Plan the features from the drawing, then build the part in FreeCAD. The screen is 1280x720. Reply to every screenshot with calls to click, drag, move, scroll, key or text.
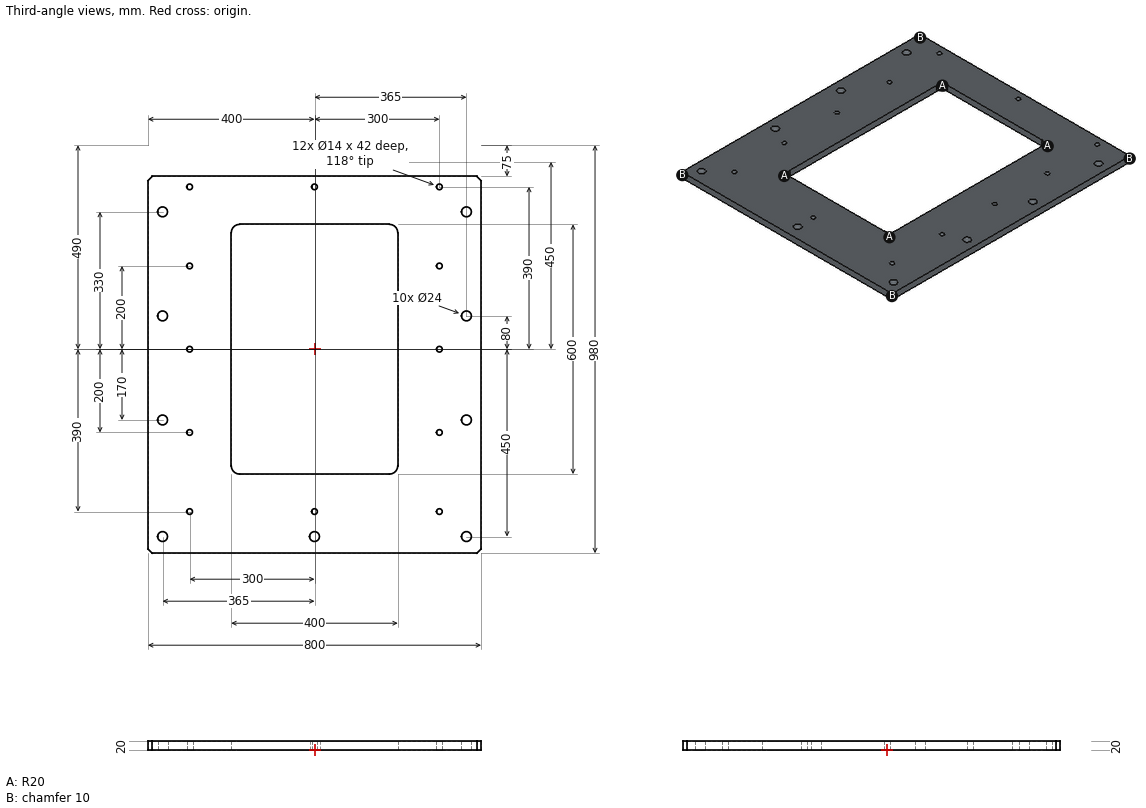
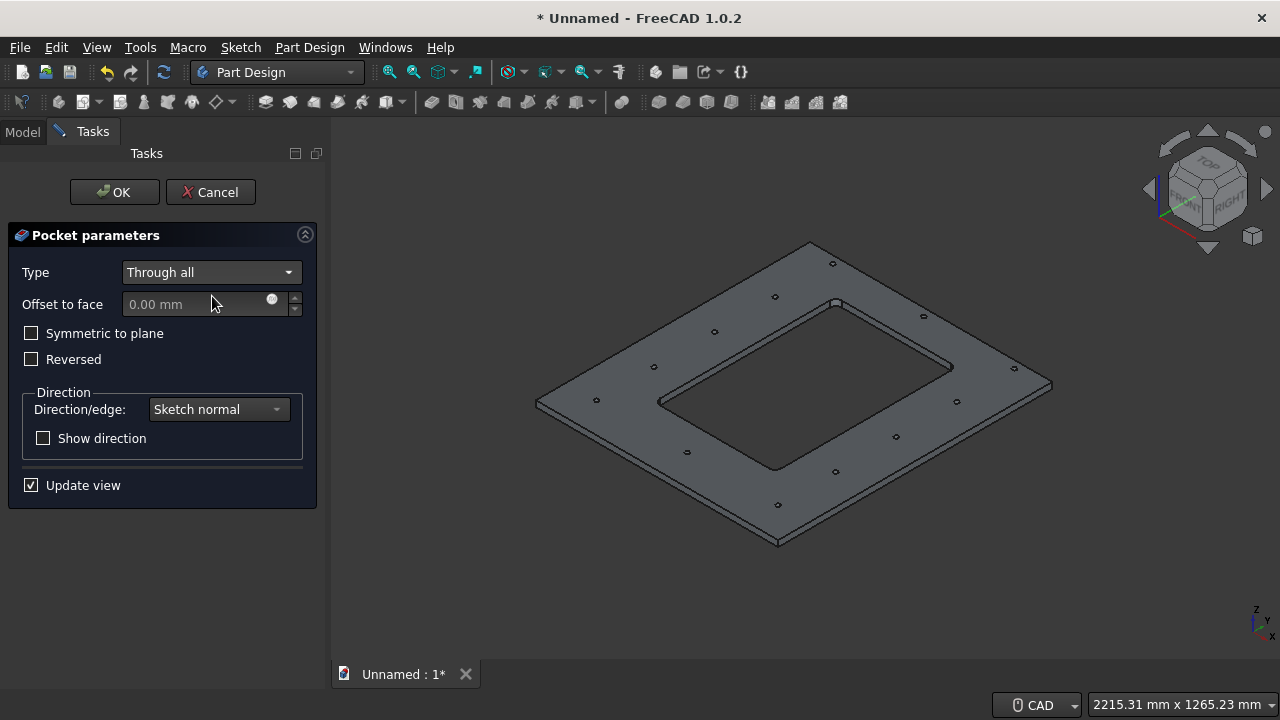
click(115, 192)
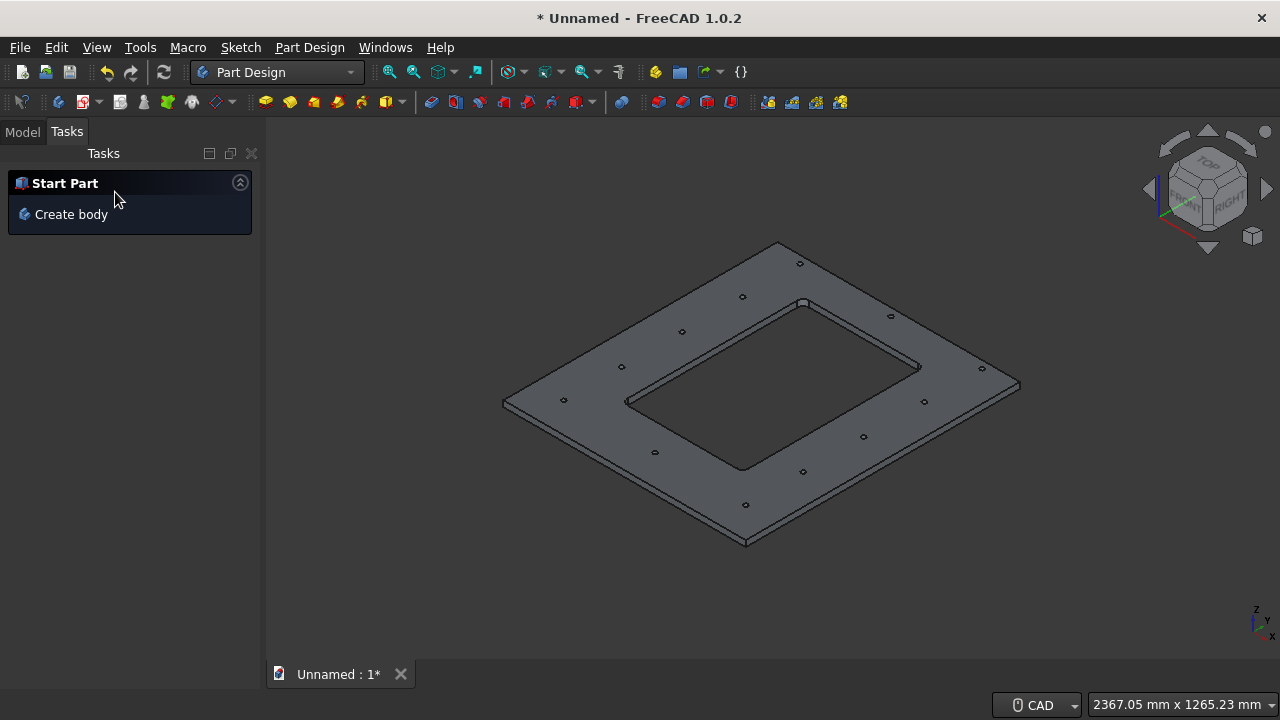
click(948, 362)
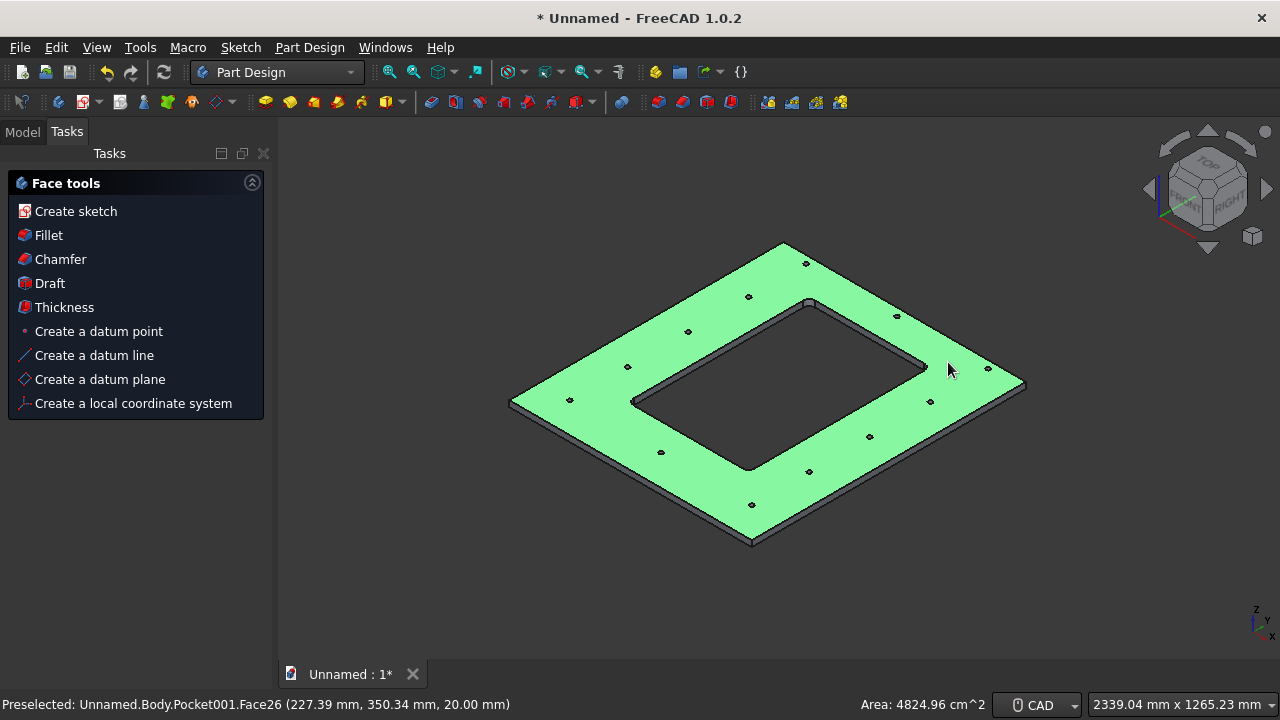
click(84, 102)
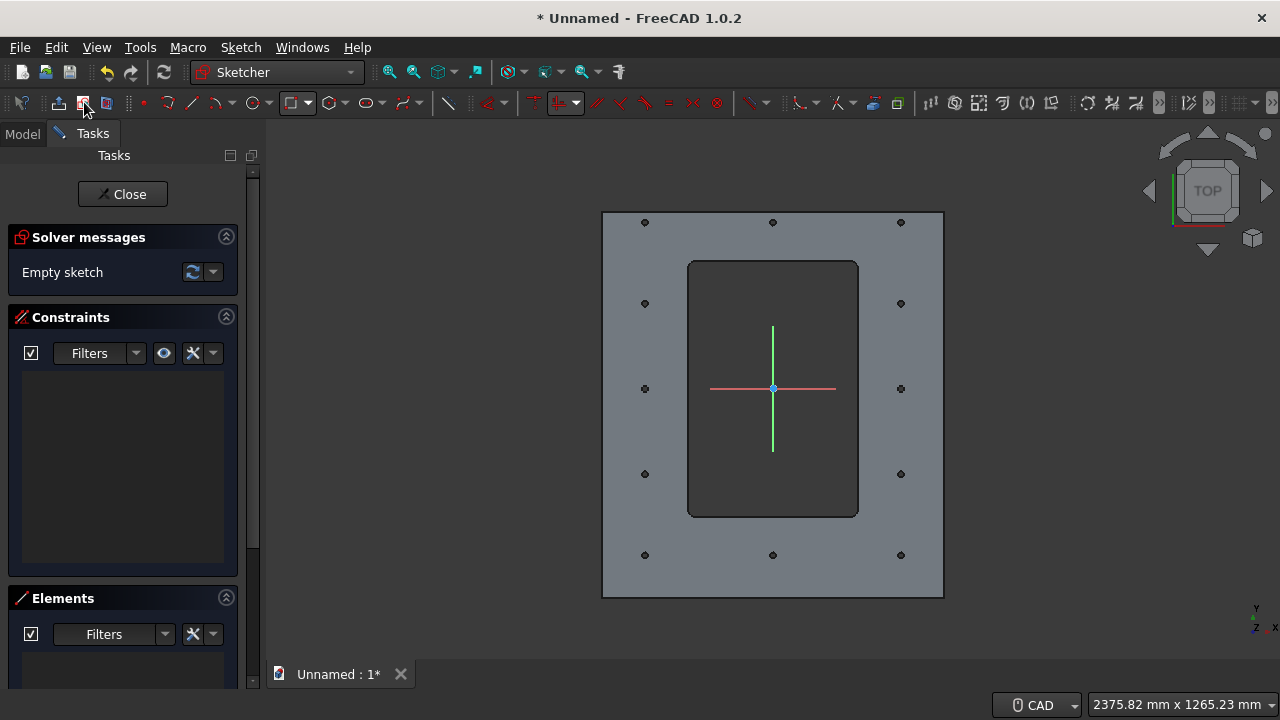
click(254, 104)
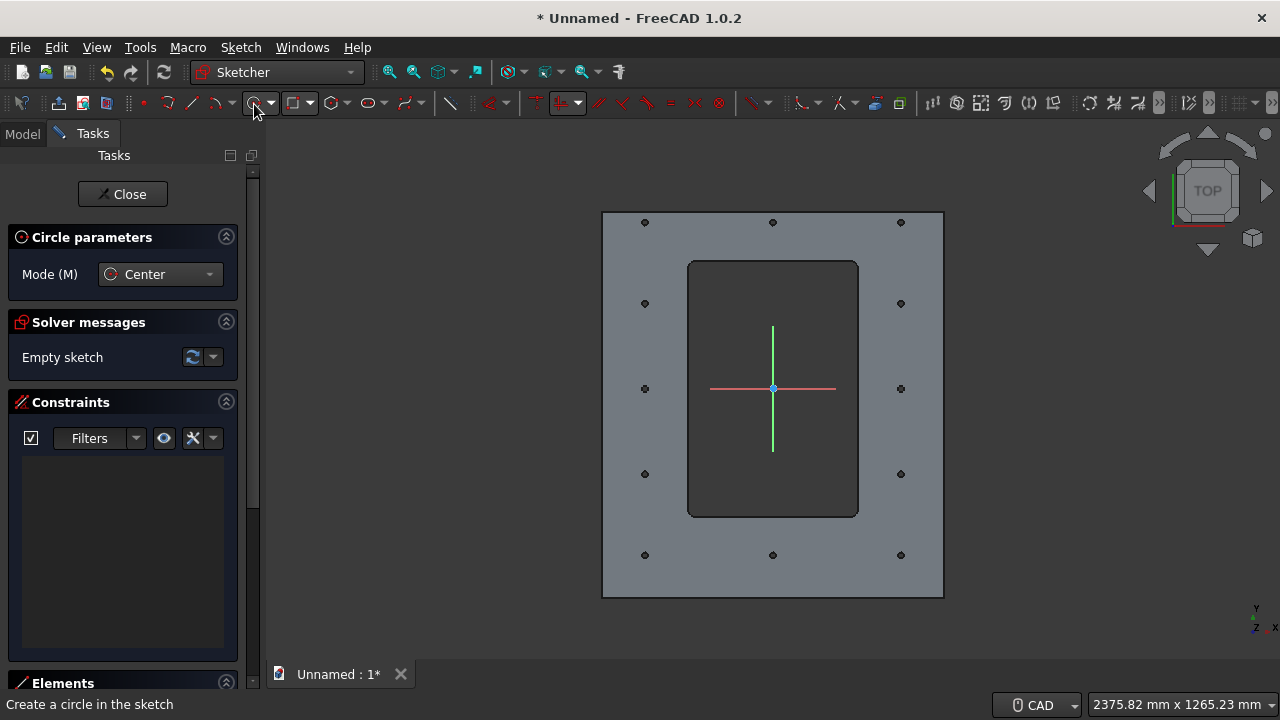
scroll(929, 355, up, 8)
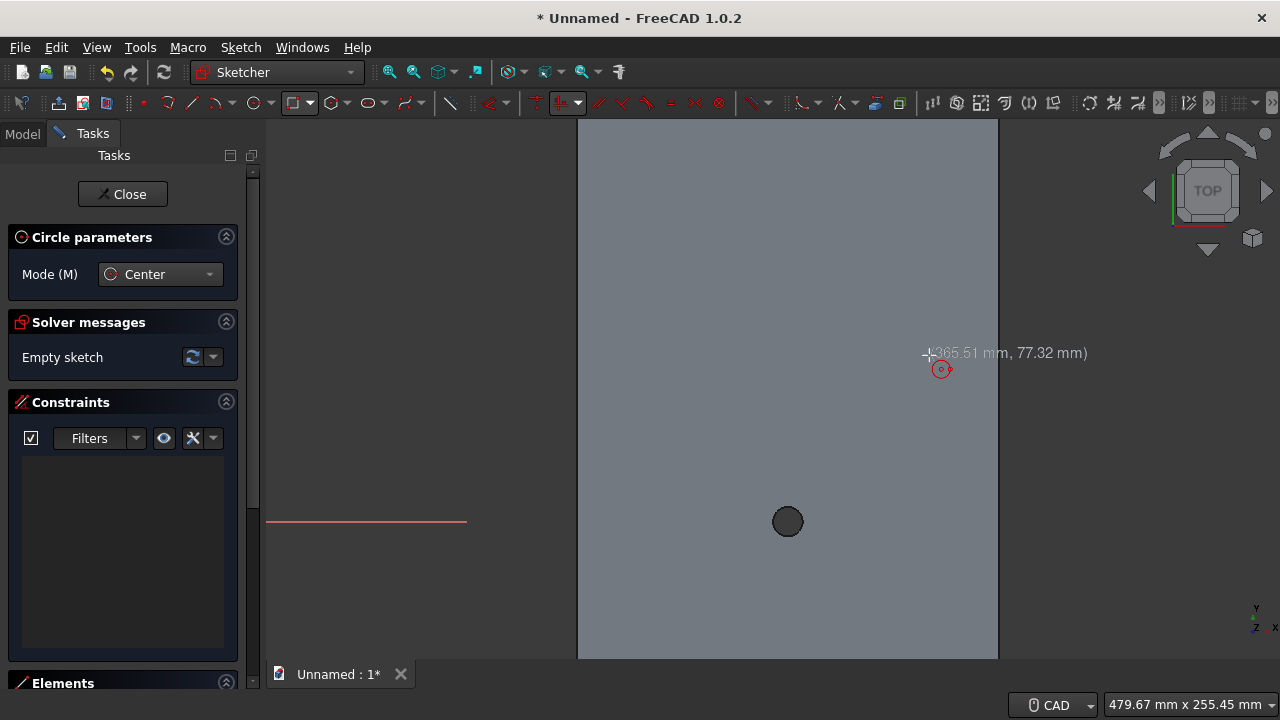
scroll(814, 363, down, 9)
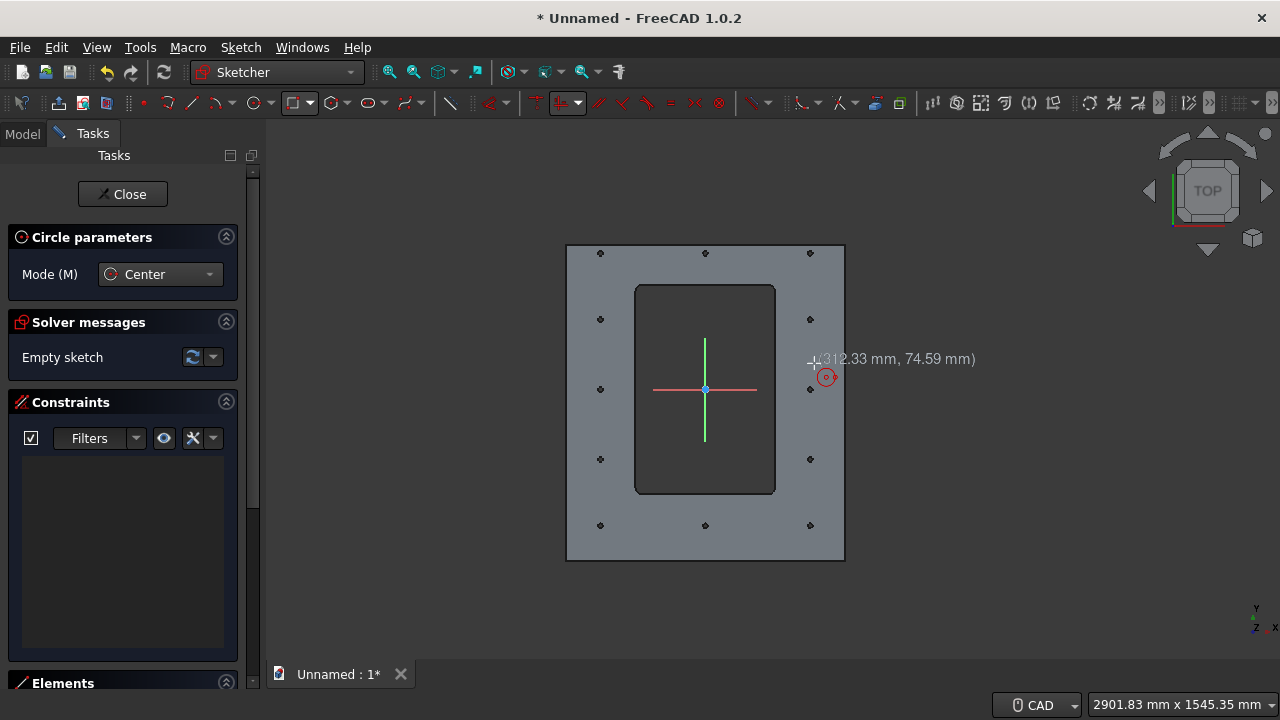
click(833, 362)
move(836, 359)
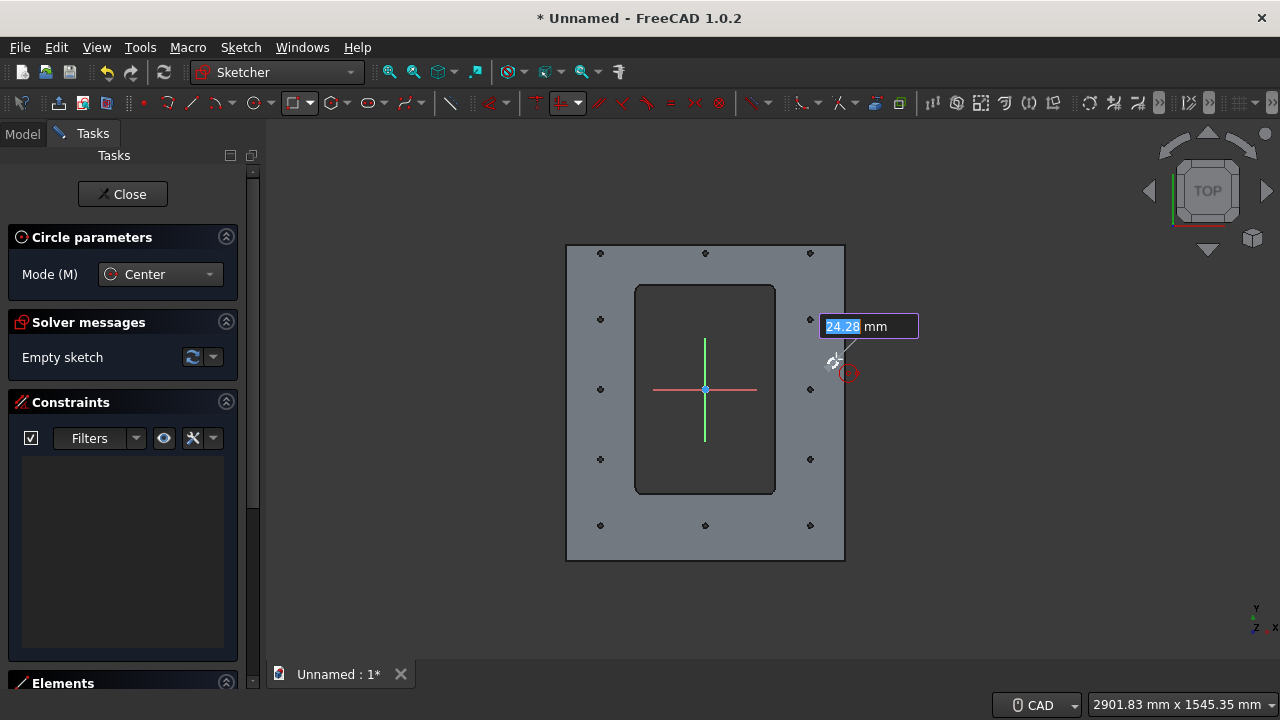
text(24)
key(Return)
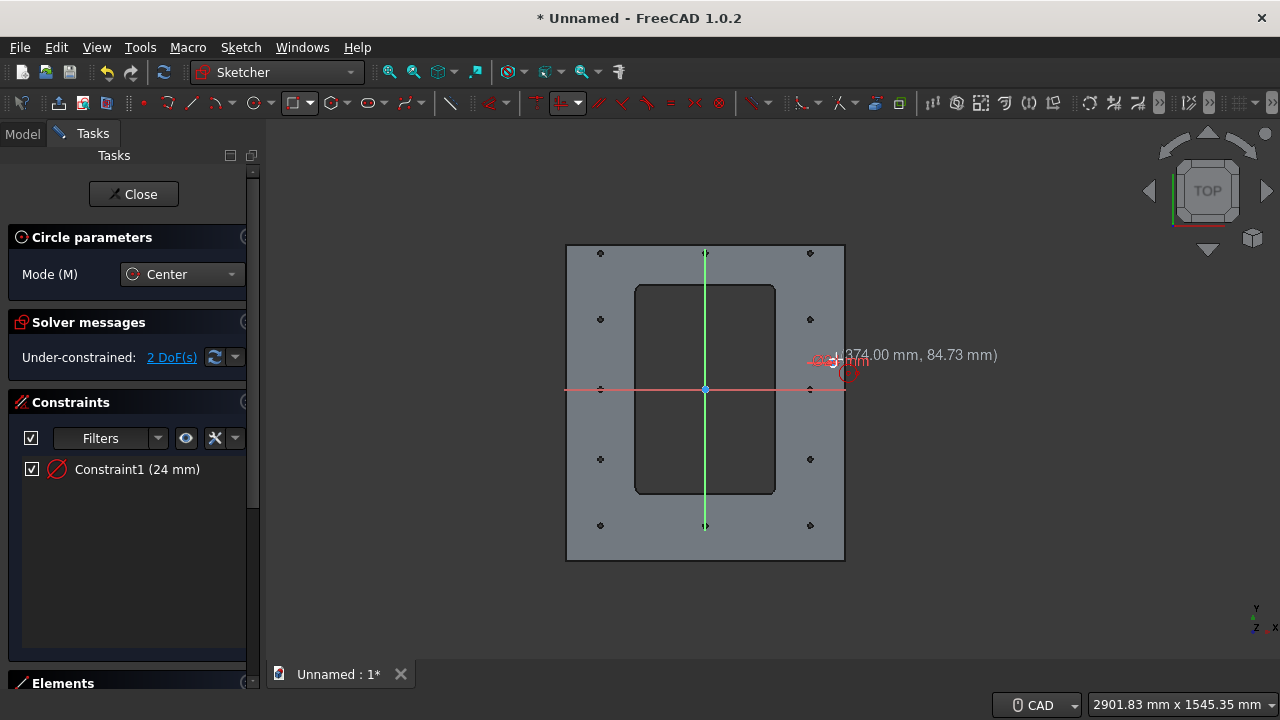
scroll(833, 547, up, 9)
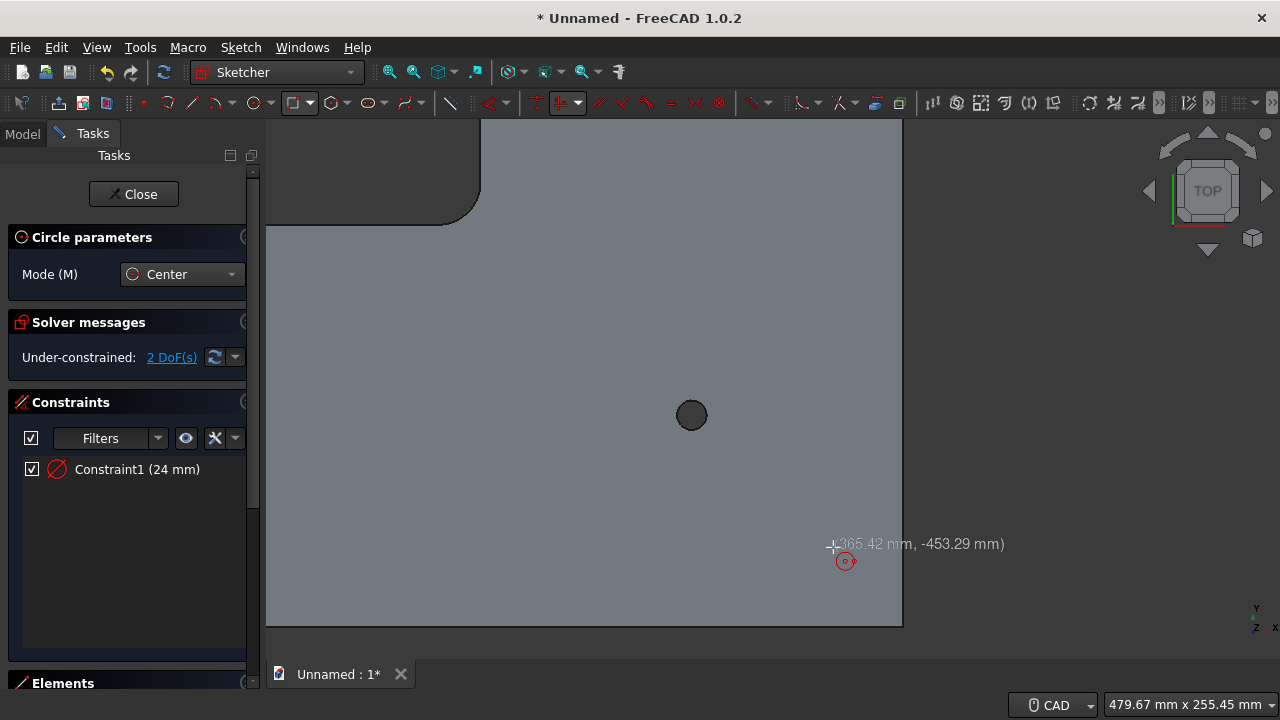
scroll(833, 547, down, 9)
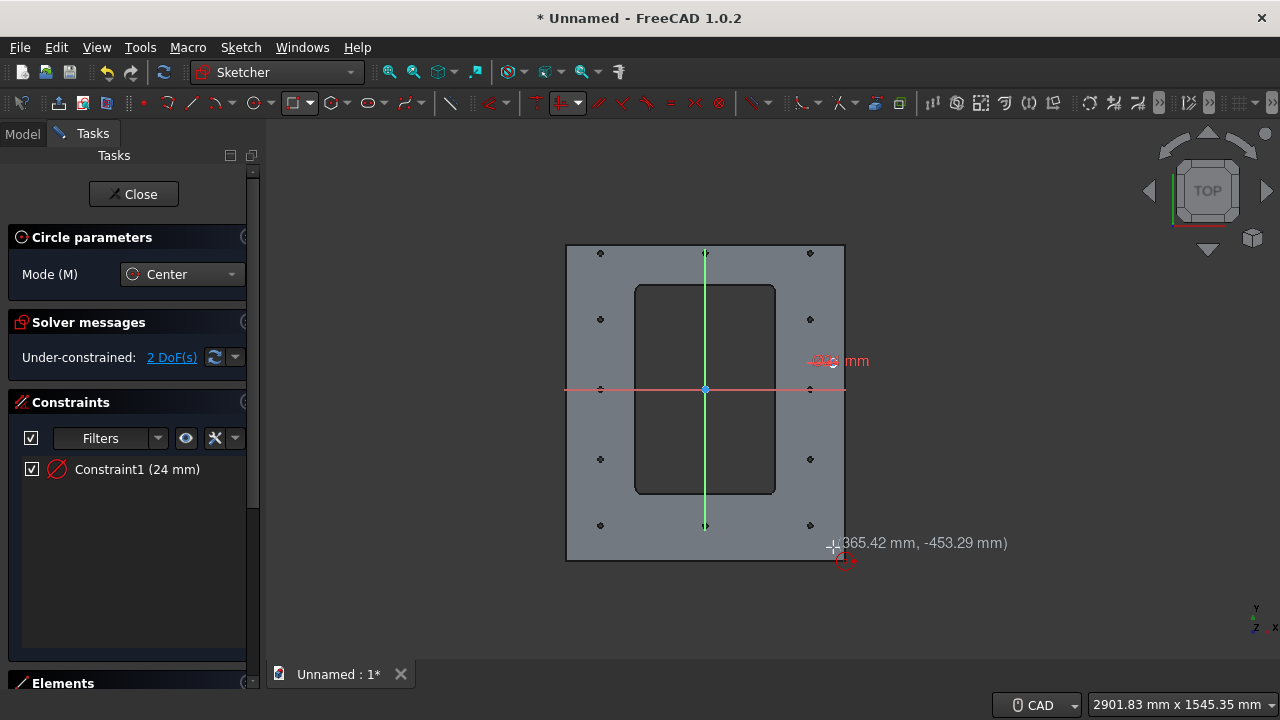
click(833, 547)
move(836, 544)